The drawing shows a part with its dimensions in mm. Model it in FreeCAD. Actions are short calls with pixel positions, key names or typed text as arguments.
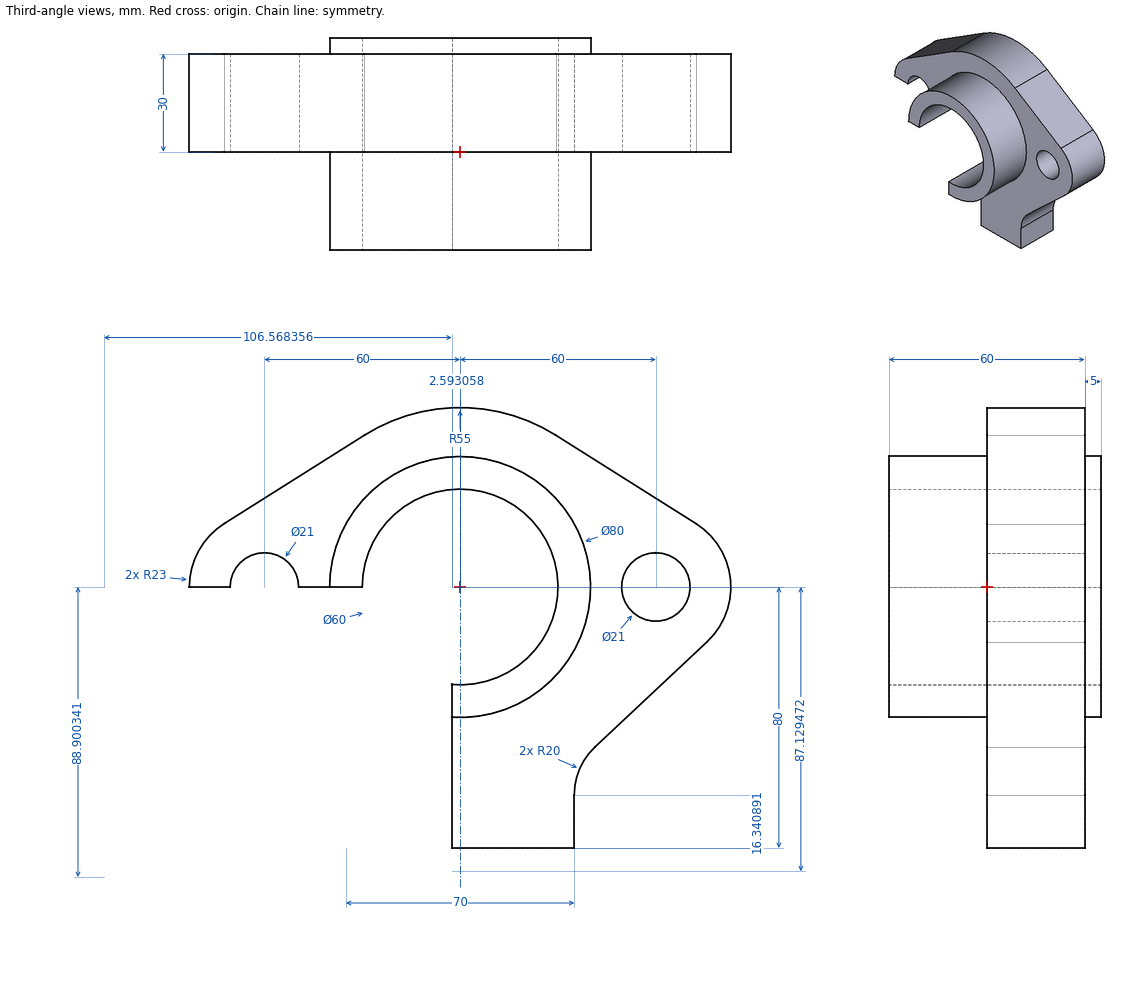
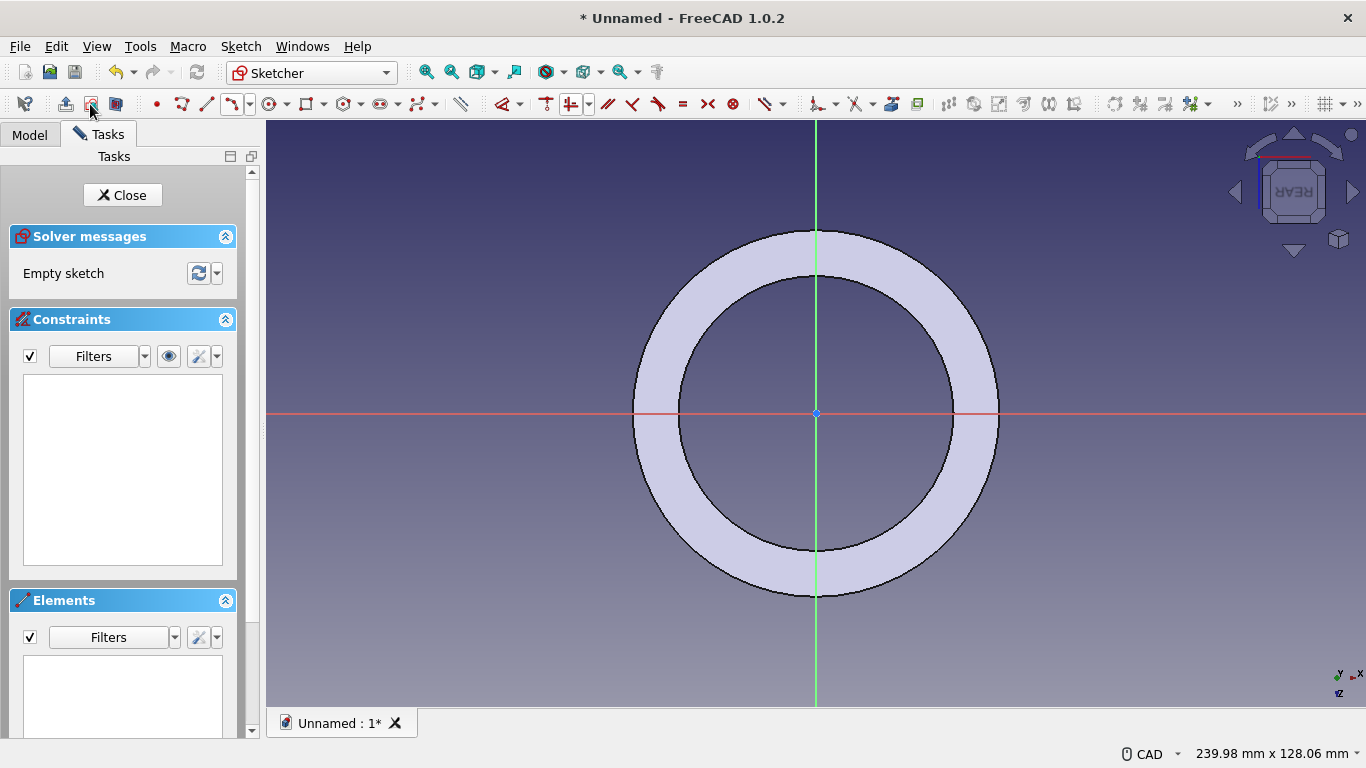
scroll(664, 483, down, 3)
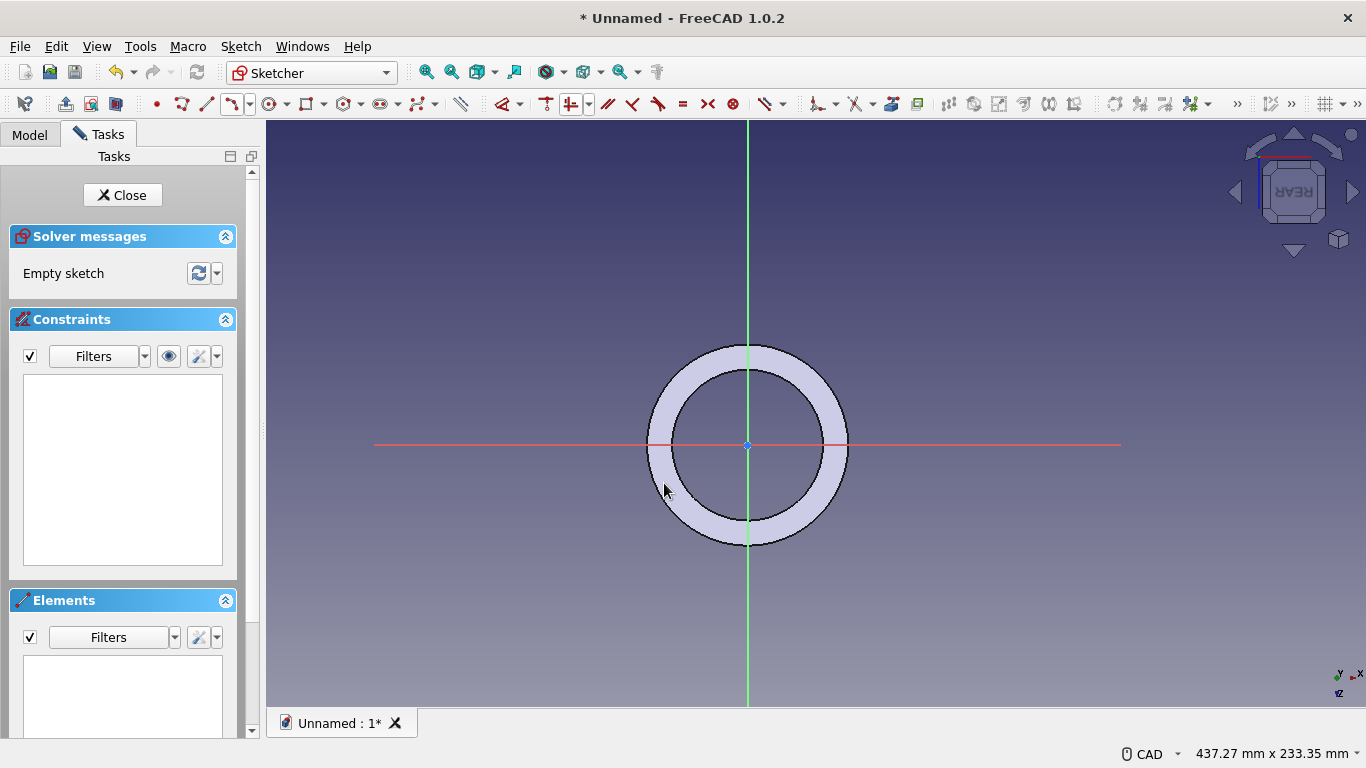
click(207, 104)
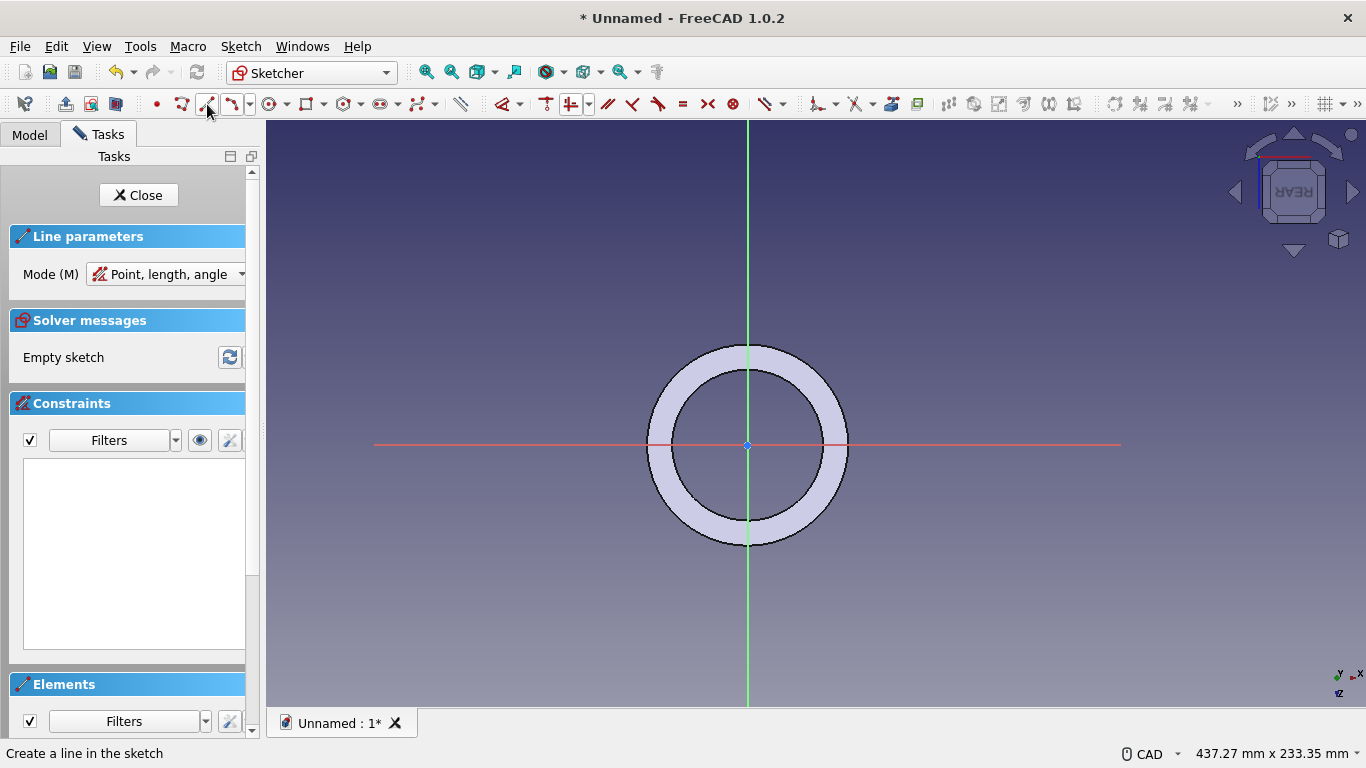
click(566, 494)
click(674, 562)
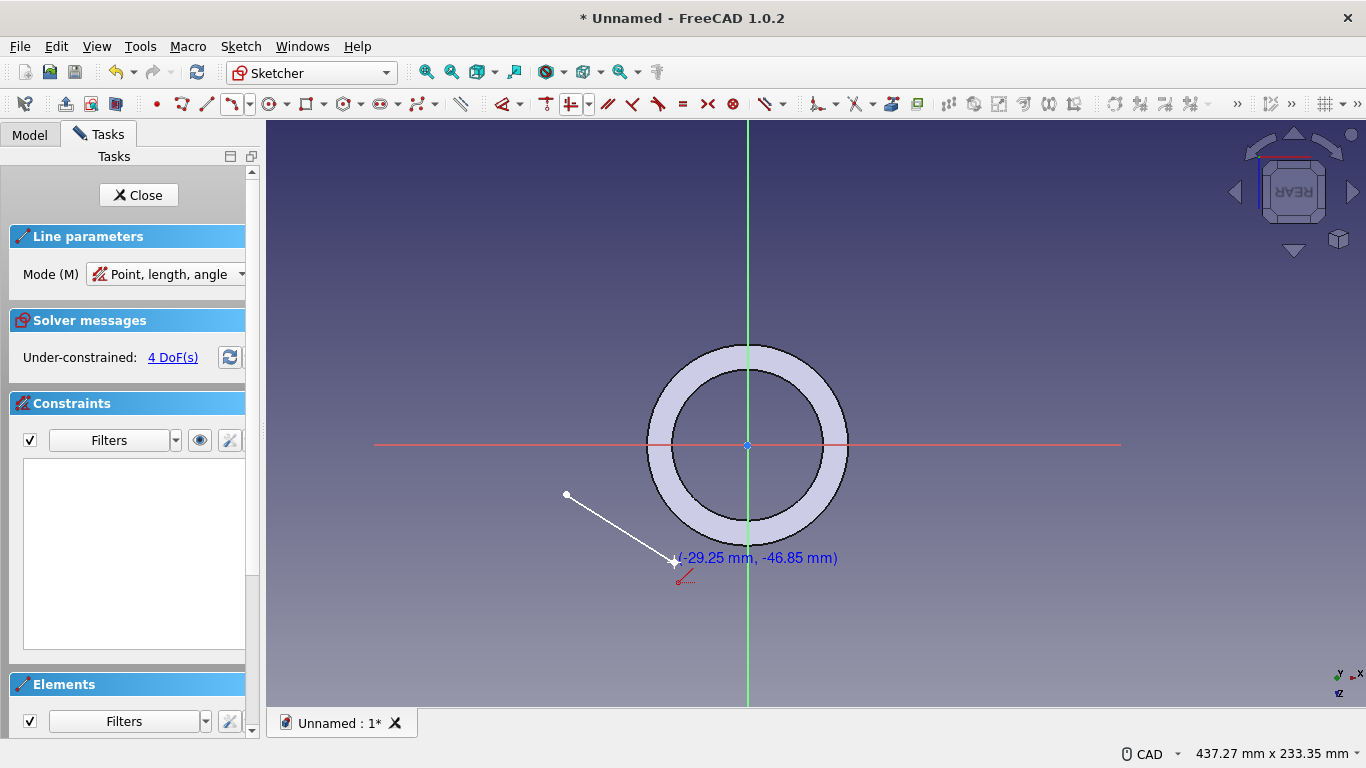
click(821, 562)
click(929, 494)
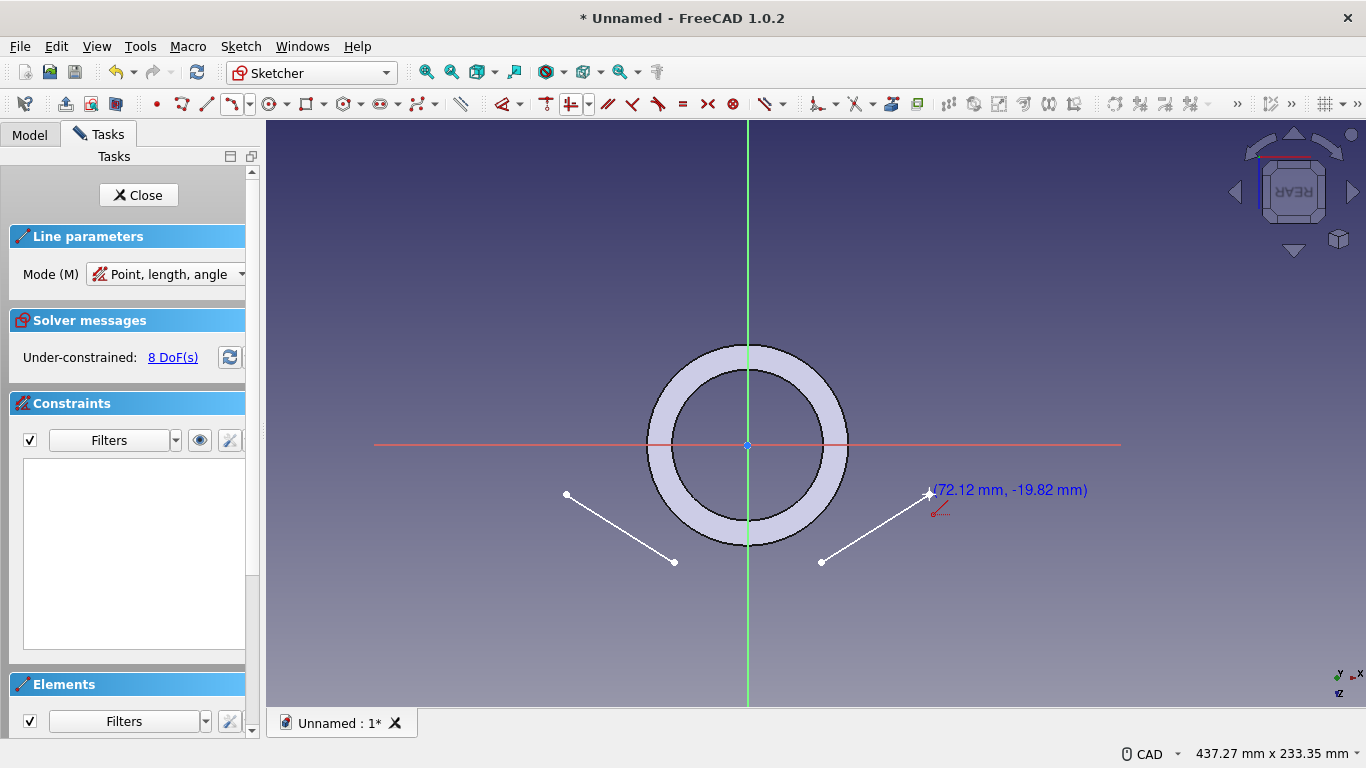
click(938, 403)
click(852, 322)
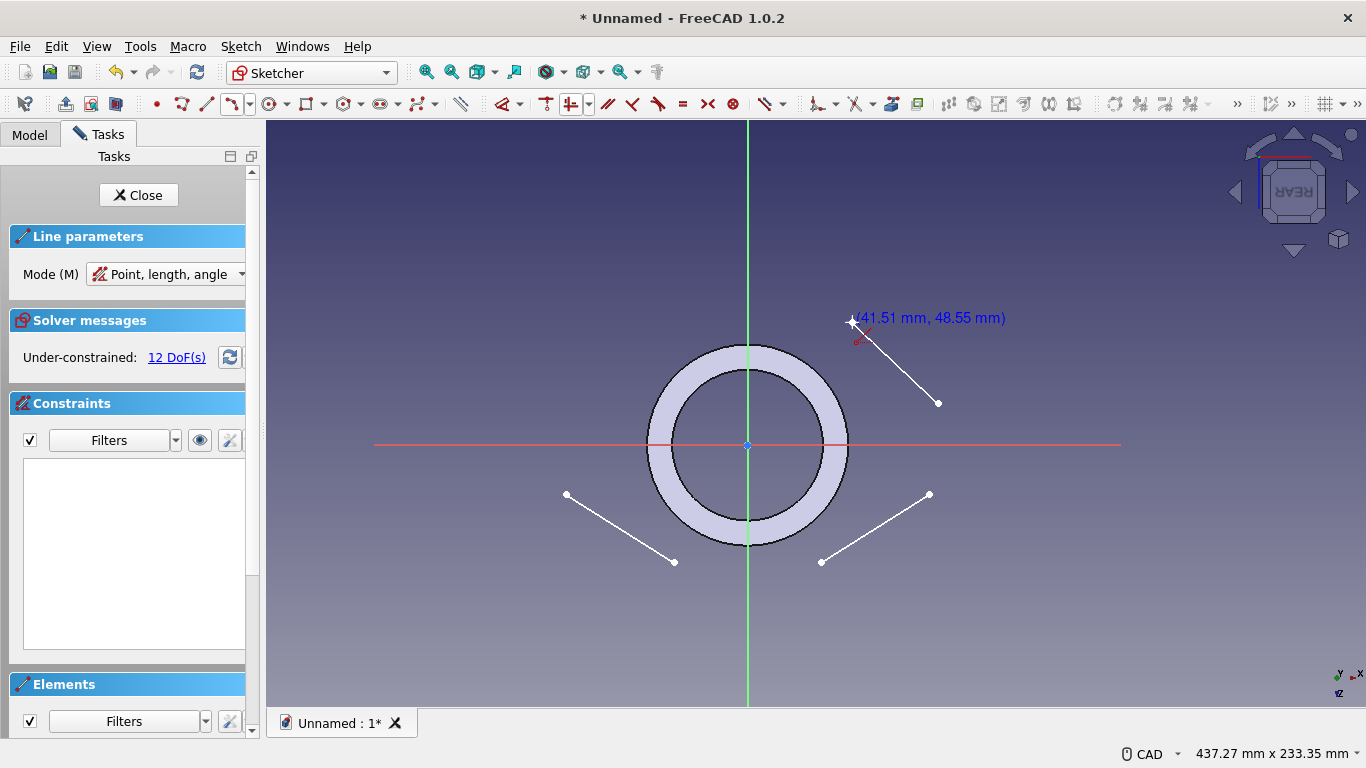
click(182, 104)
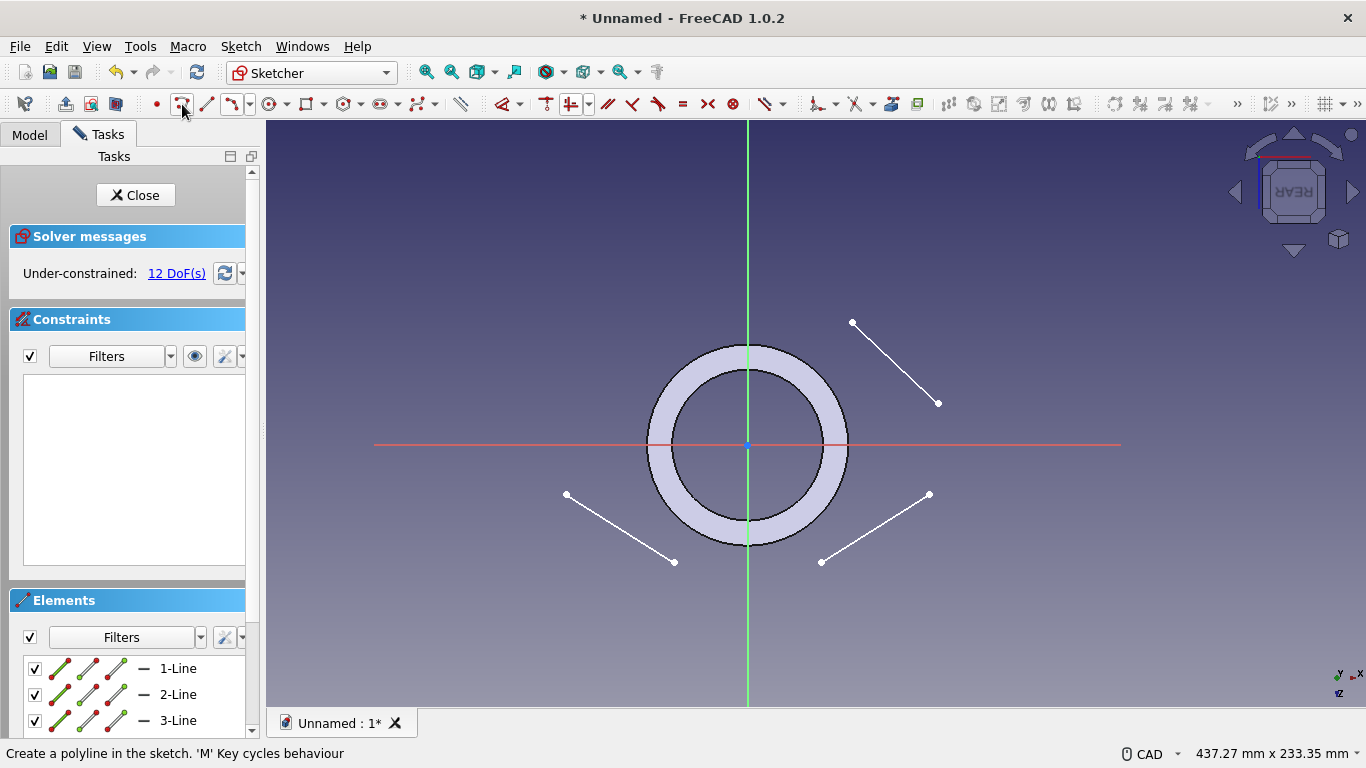
click(836, 285)
click(836, 244)
click(660, 244)
click(660, 285)
right_click(660, 285)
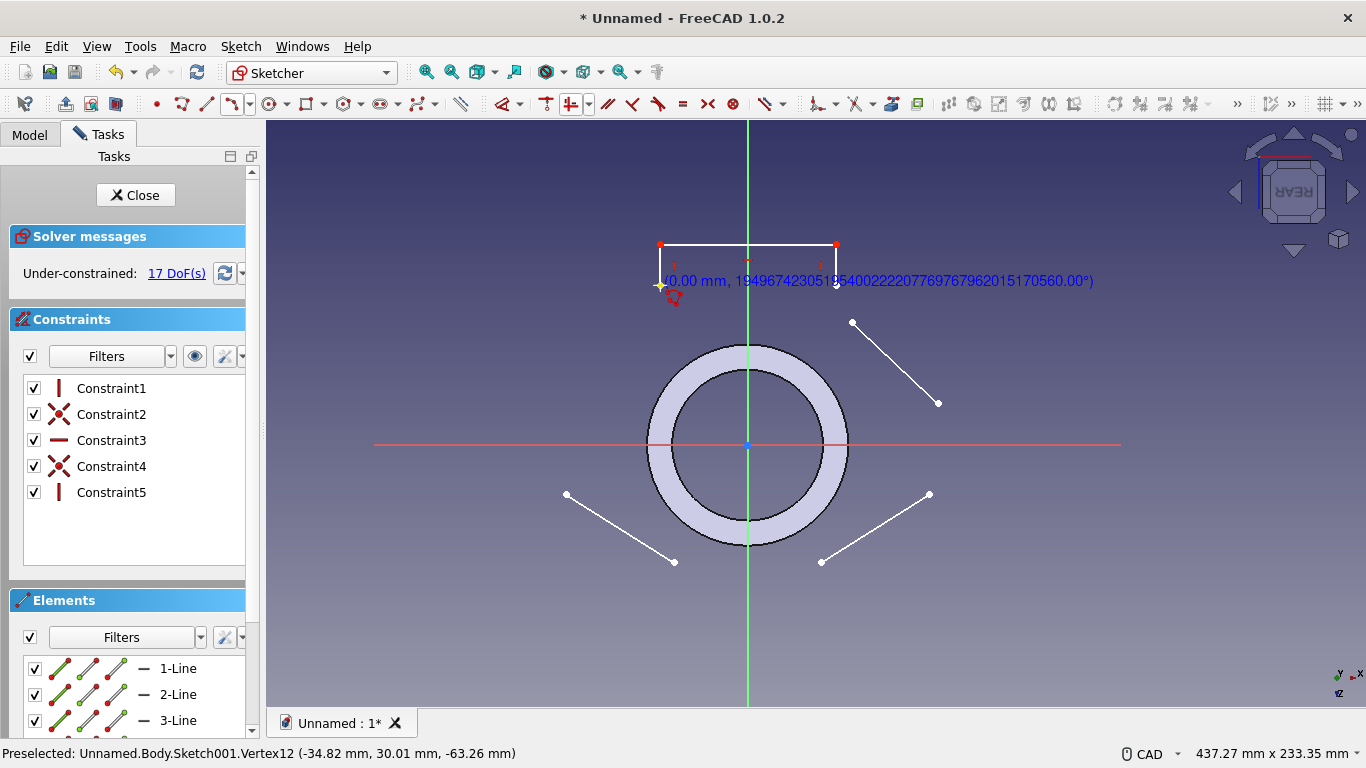
click(207, 104)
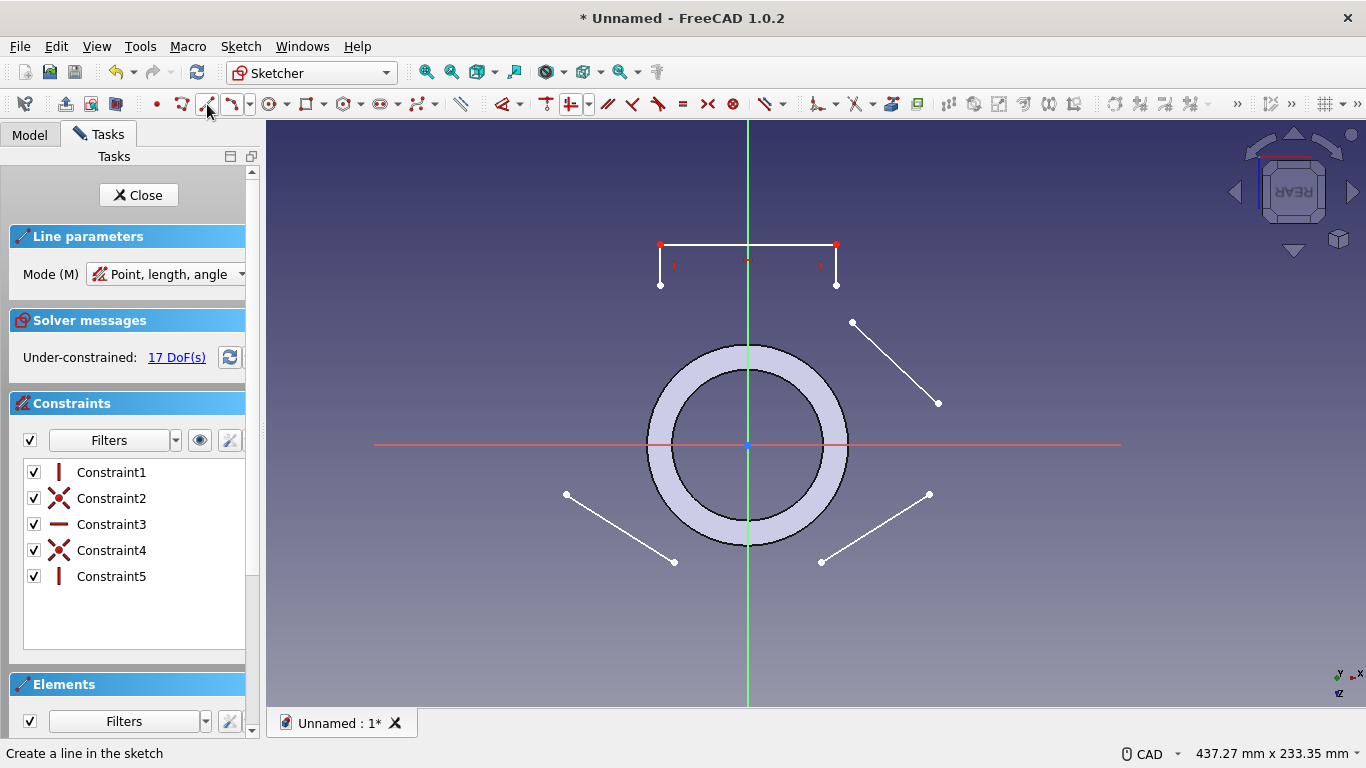
click(644, 322)
click(557, 403)